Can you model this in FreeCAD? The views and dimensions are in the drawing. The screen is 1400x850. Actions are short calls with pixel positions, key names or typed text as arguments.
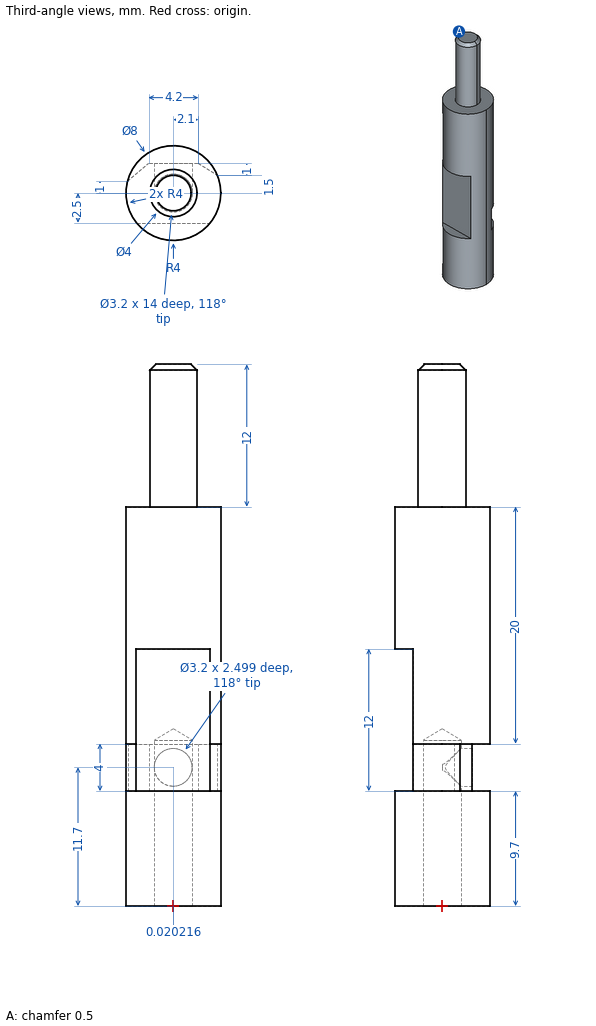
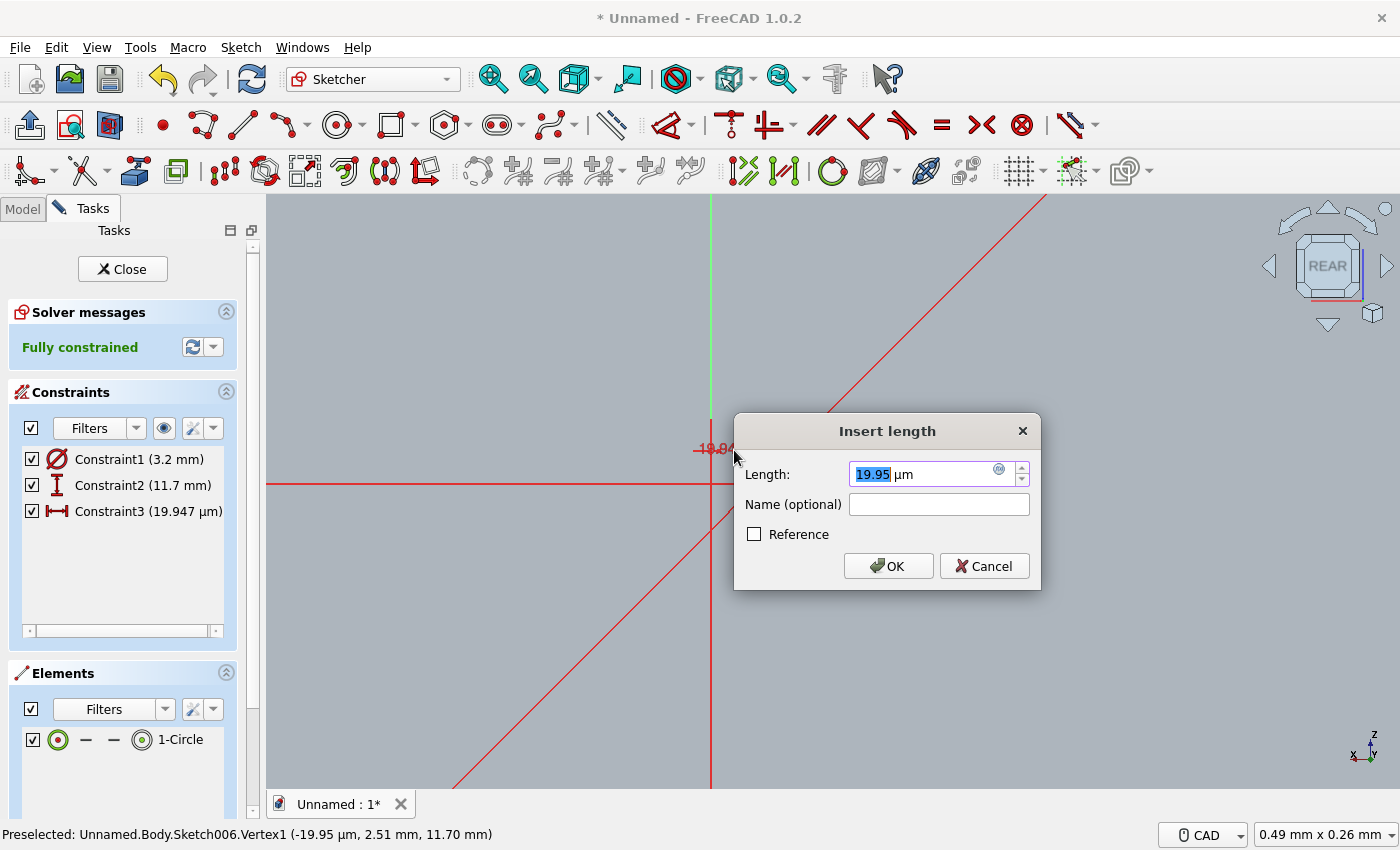
key(ctrl+a)
text(0.020216 mm)
key(Return)
key(Escape)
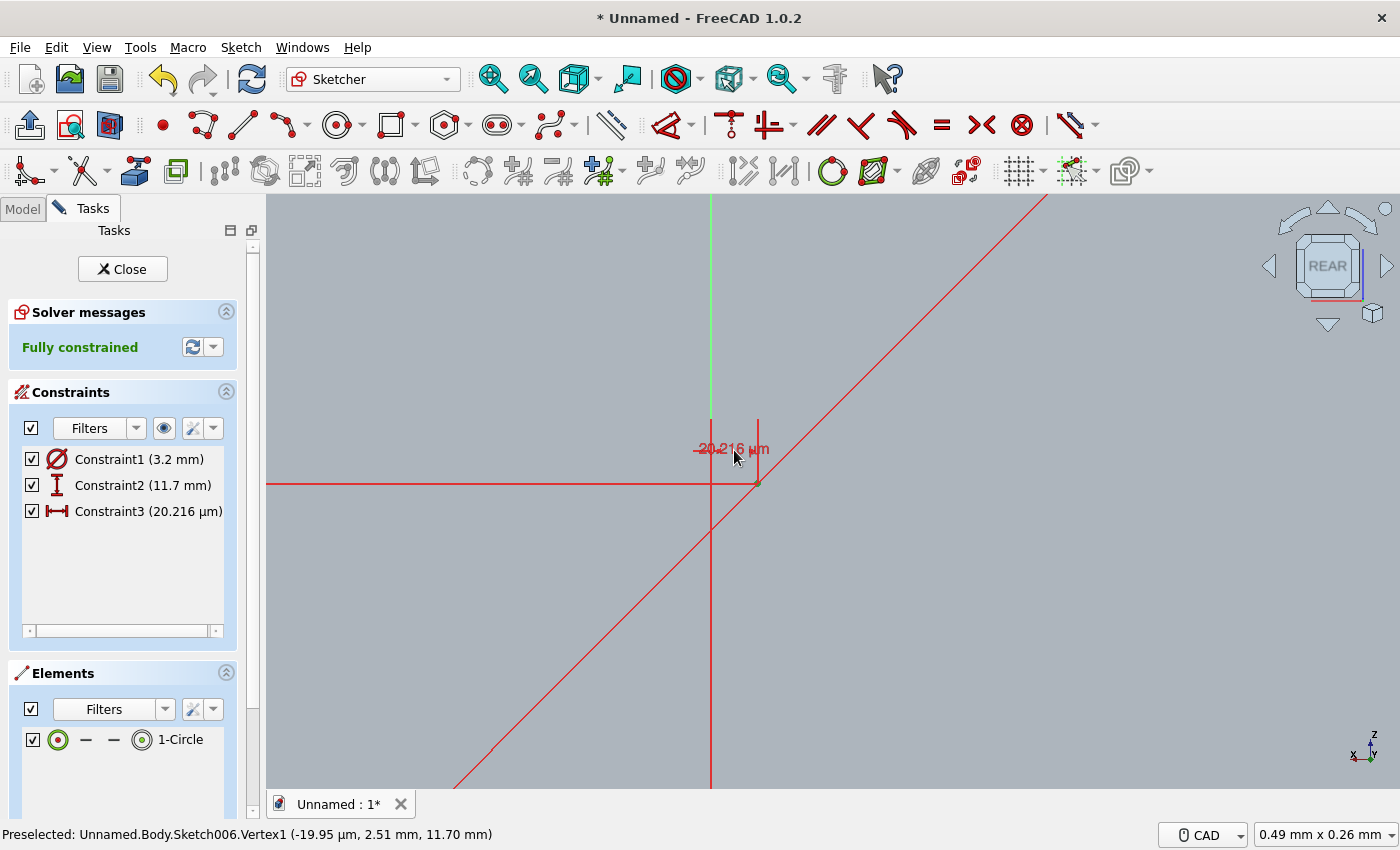
click(123, 269)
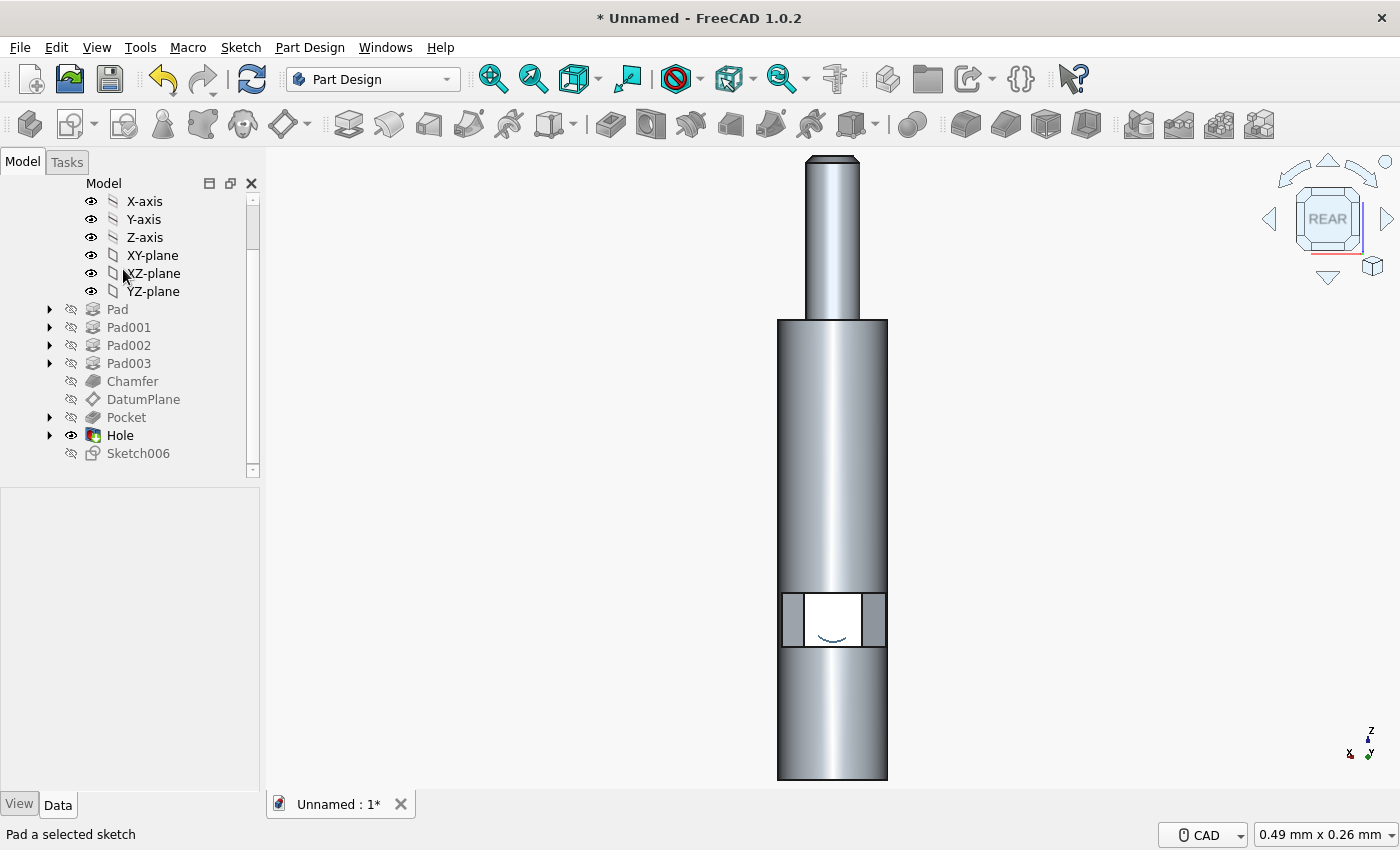
click(652, 124)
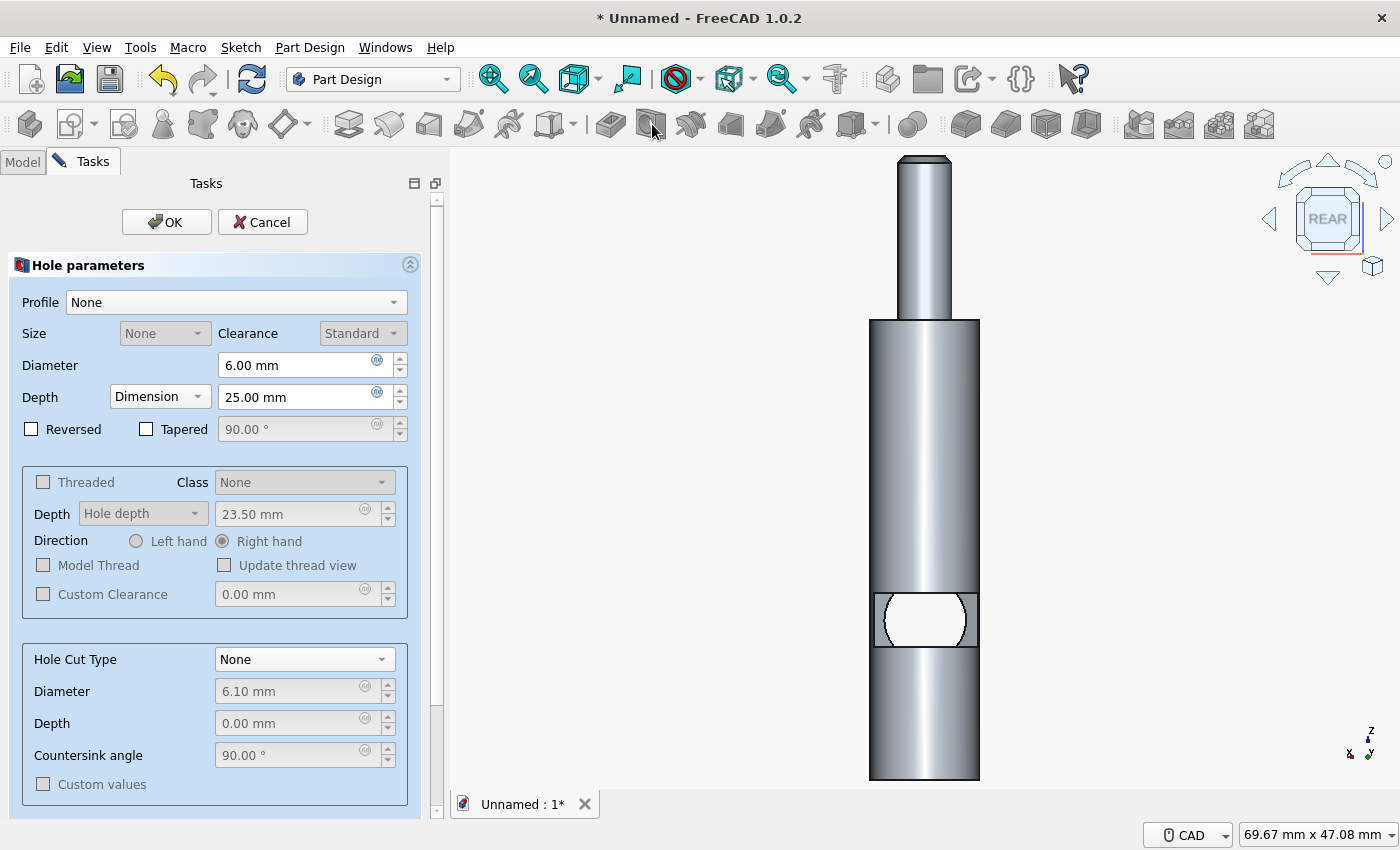
triple_click(305, 365)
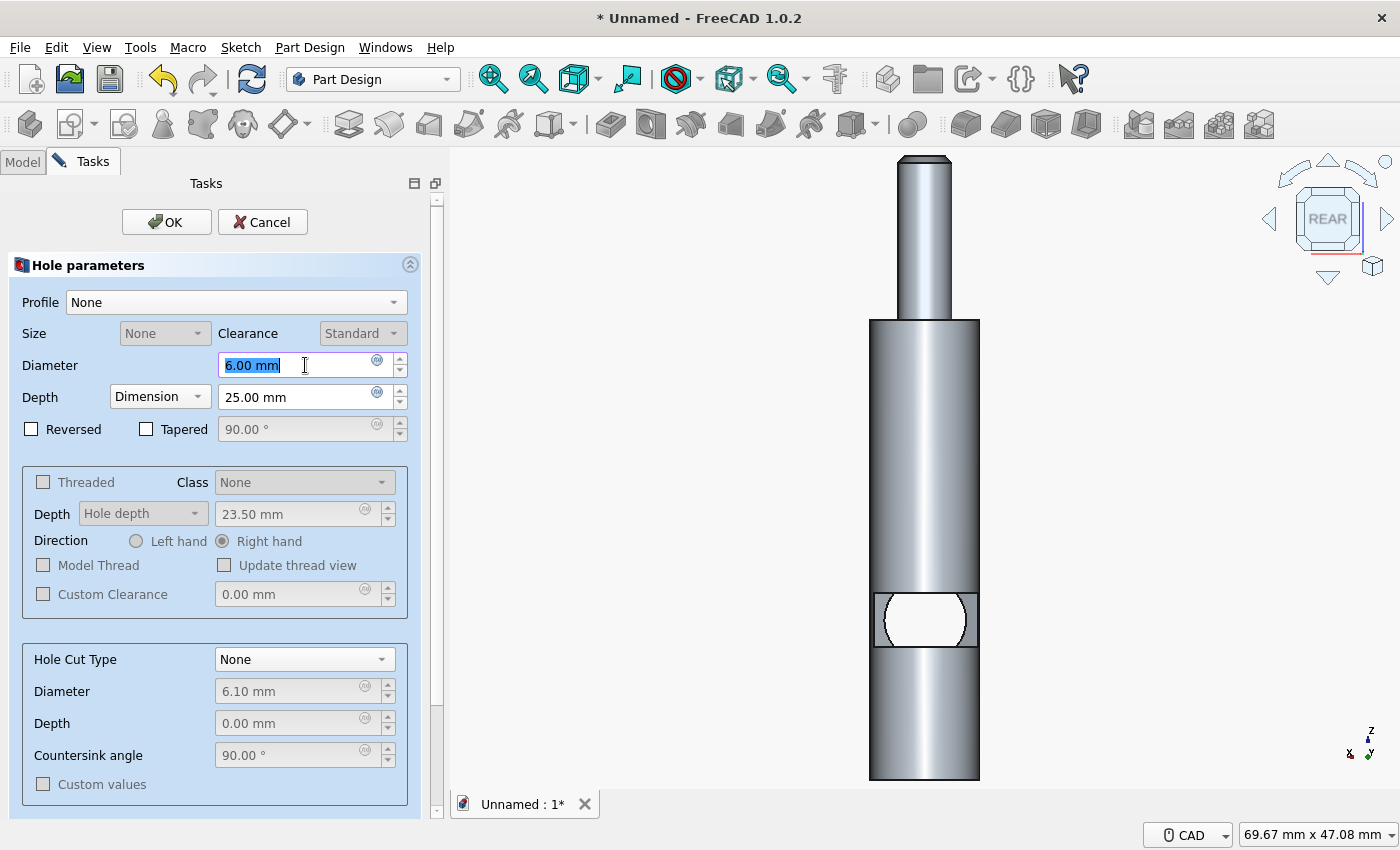
text(3.2)
key(Tab)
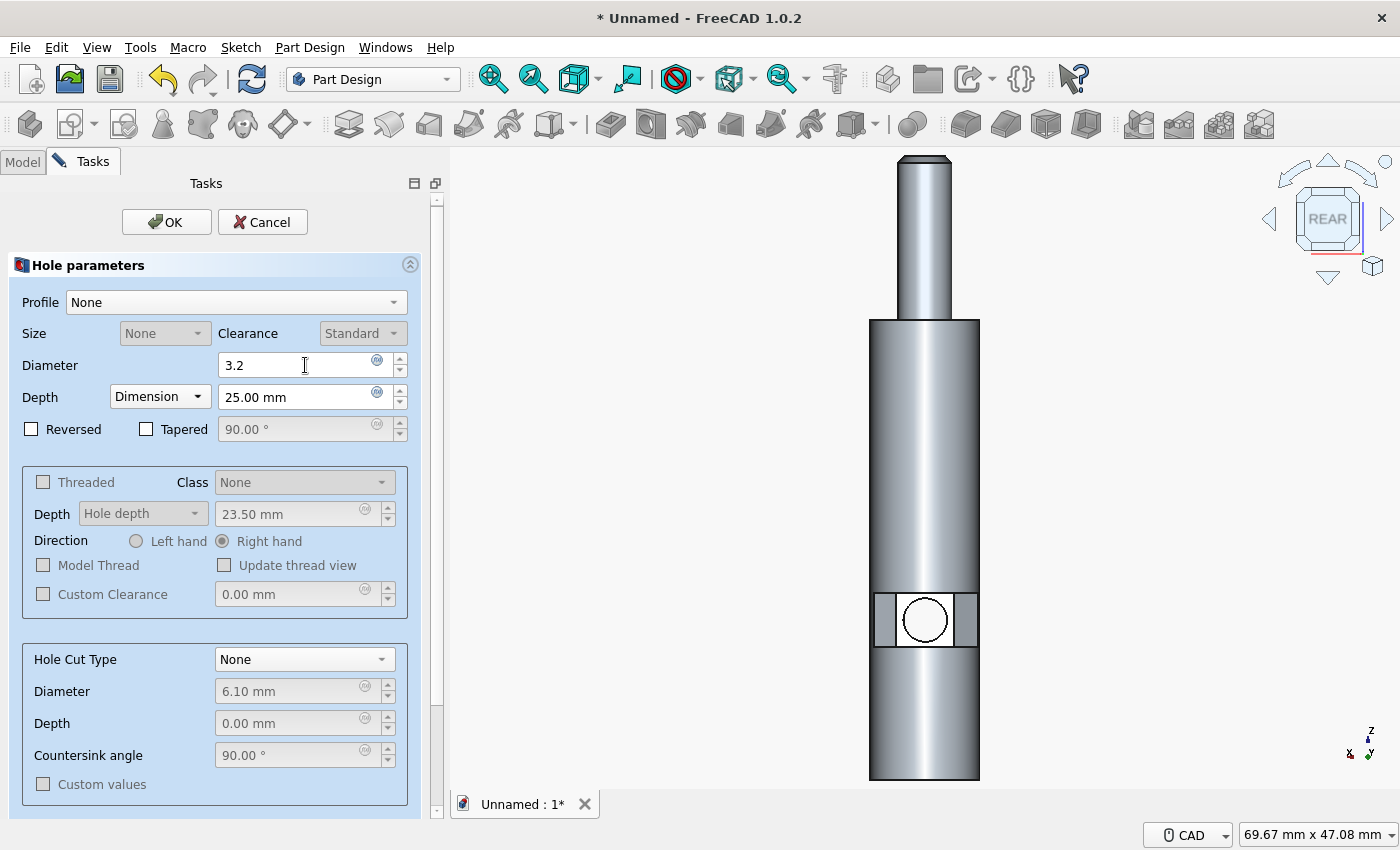
triple_click(305, 397)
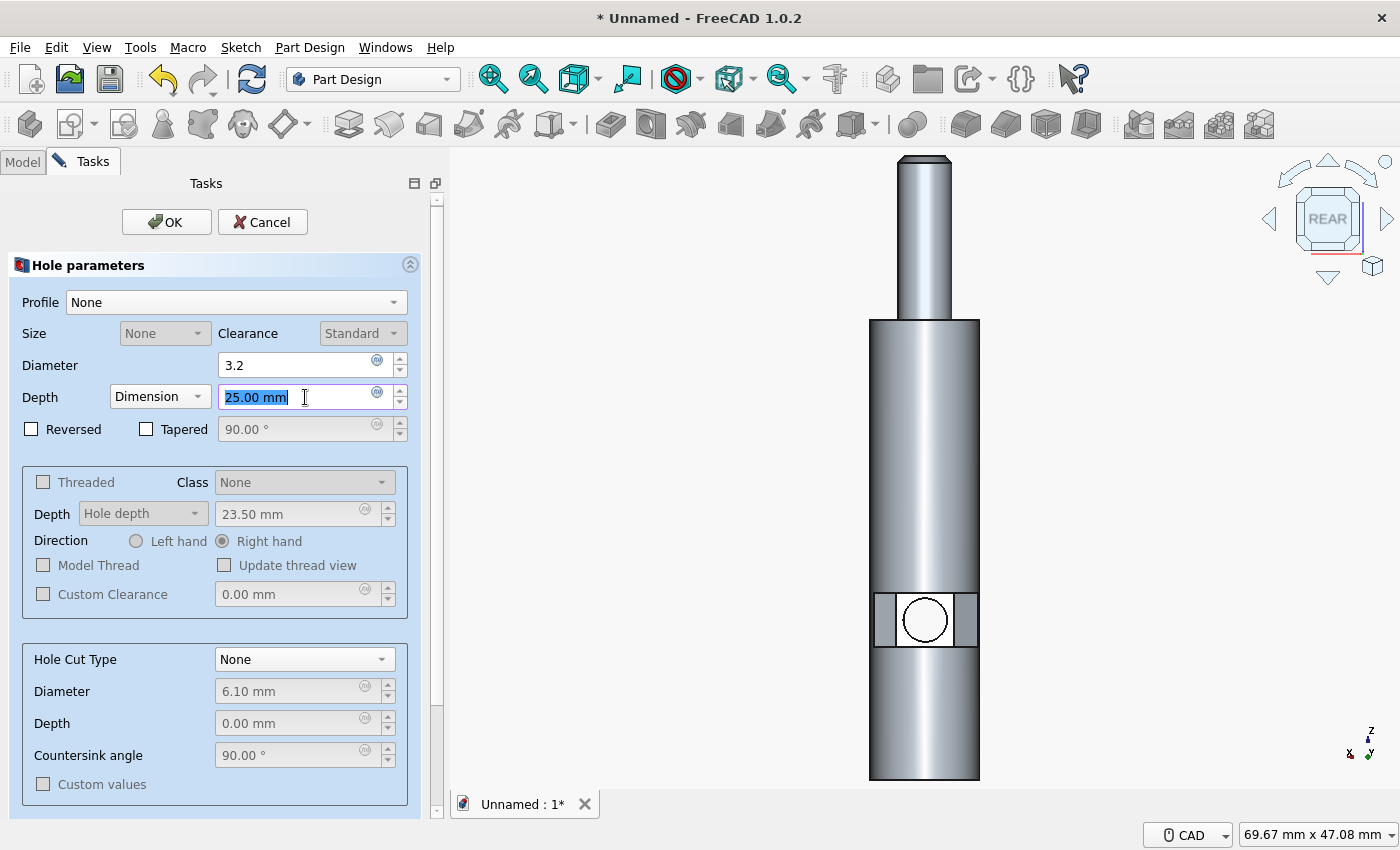
text(2.499)
key(Tab)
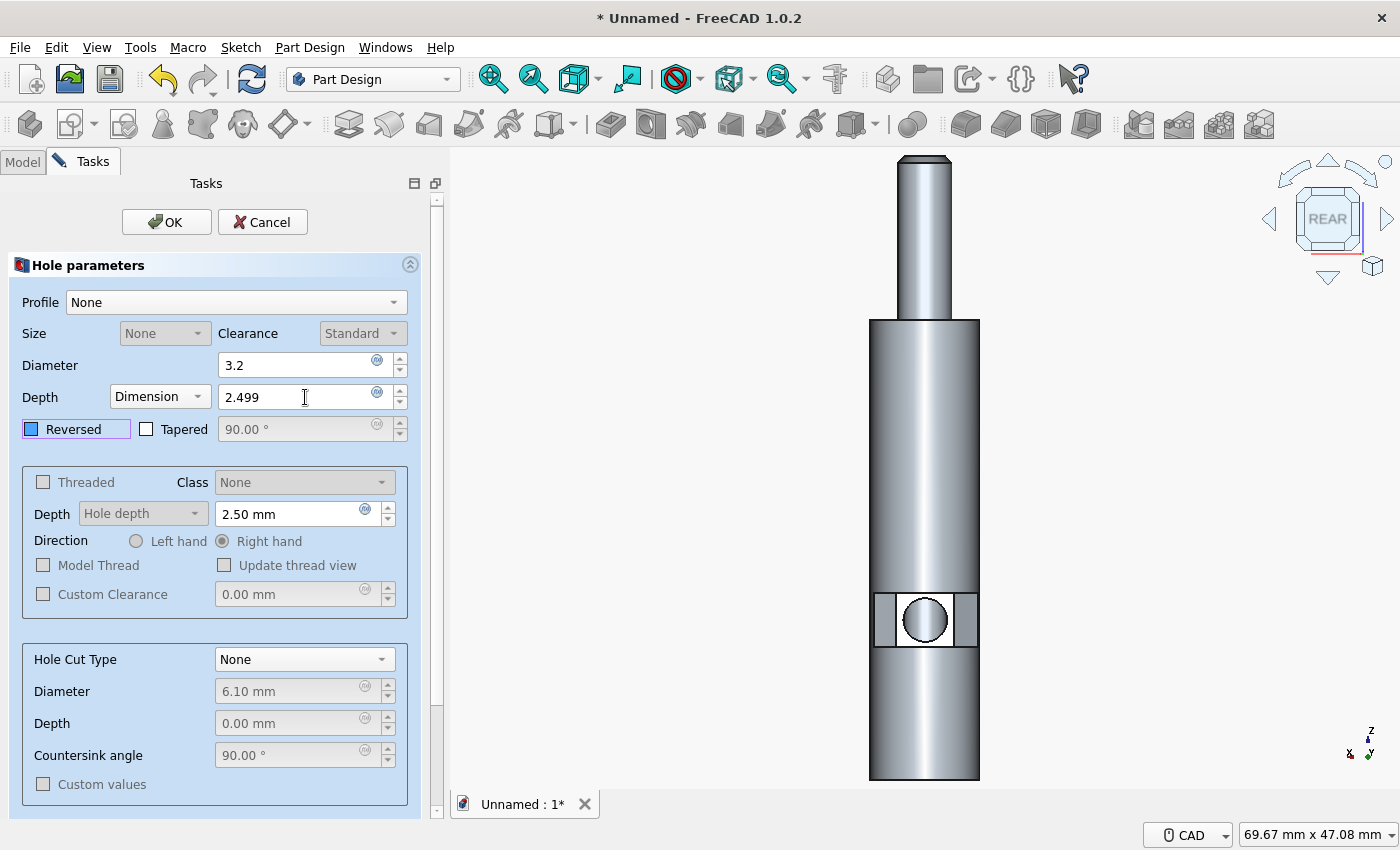
click(167, 222)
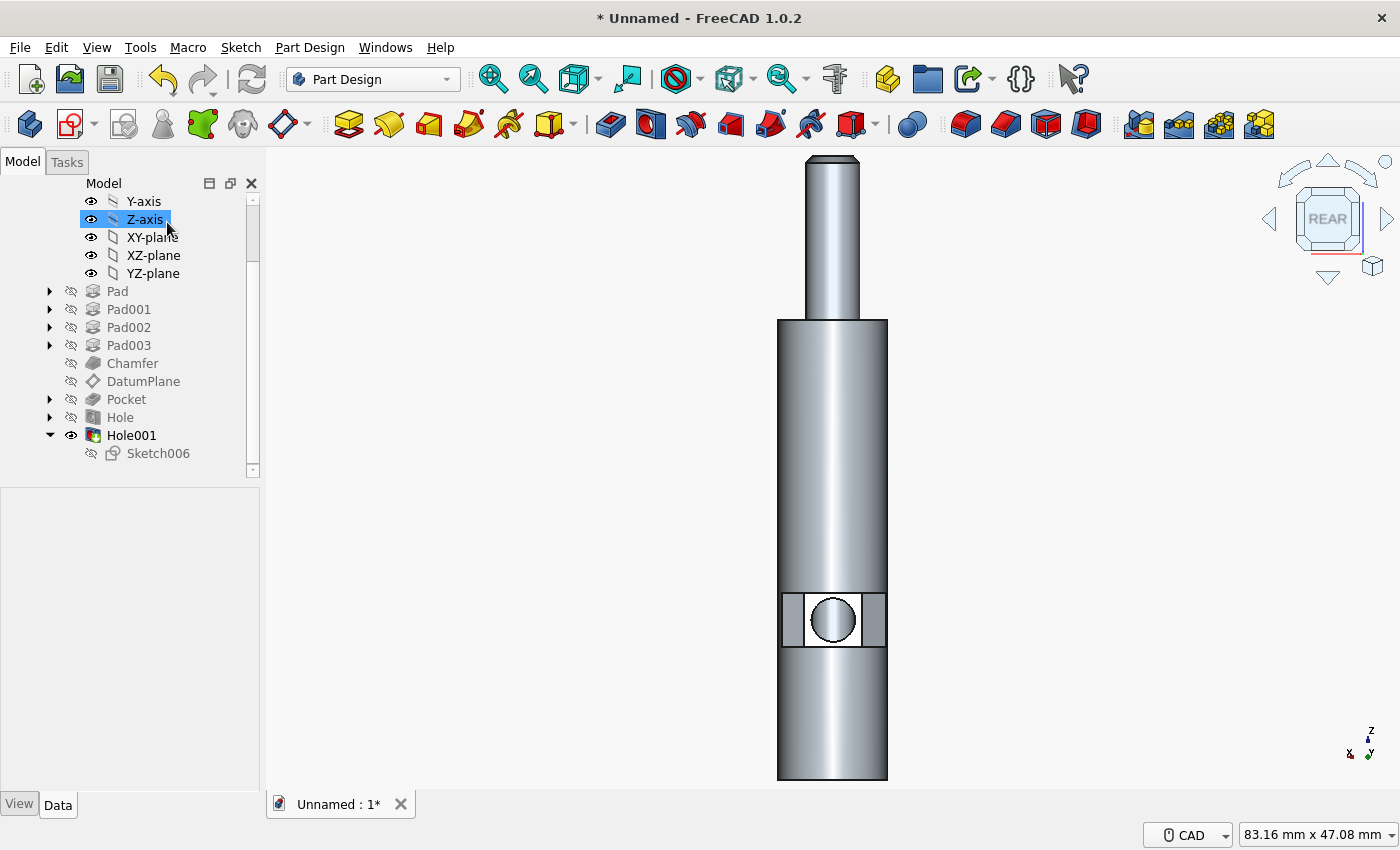
key(0)